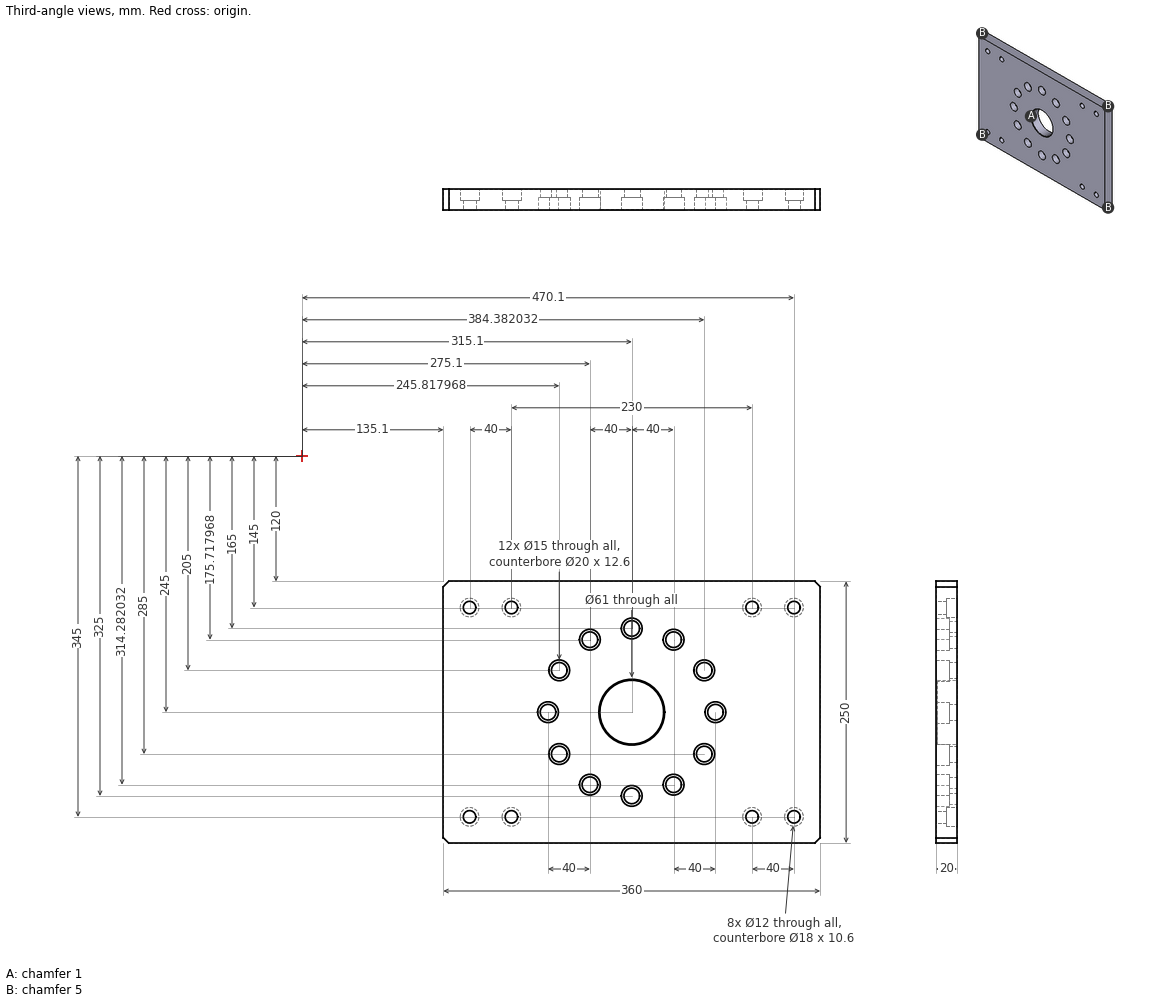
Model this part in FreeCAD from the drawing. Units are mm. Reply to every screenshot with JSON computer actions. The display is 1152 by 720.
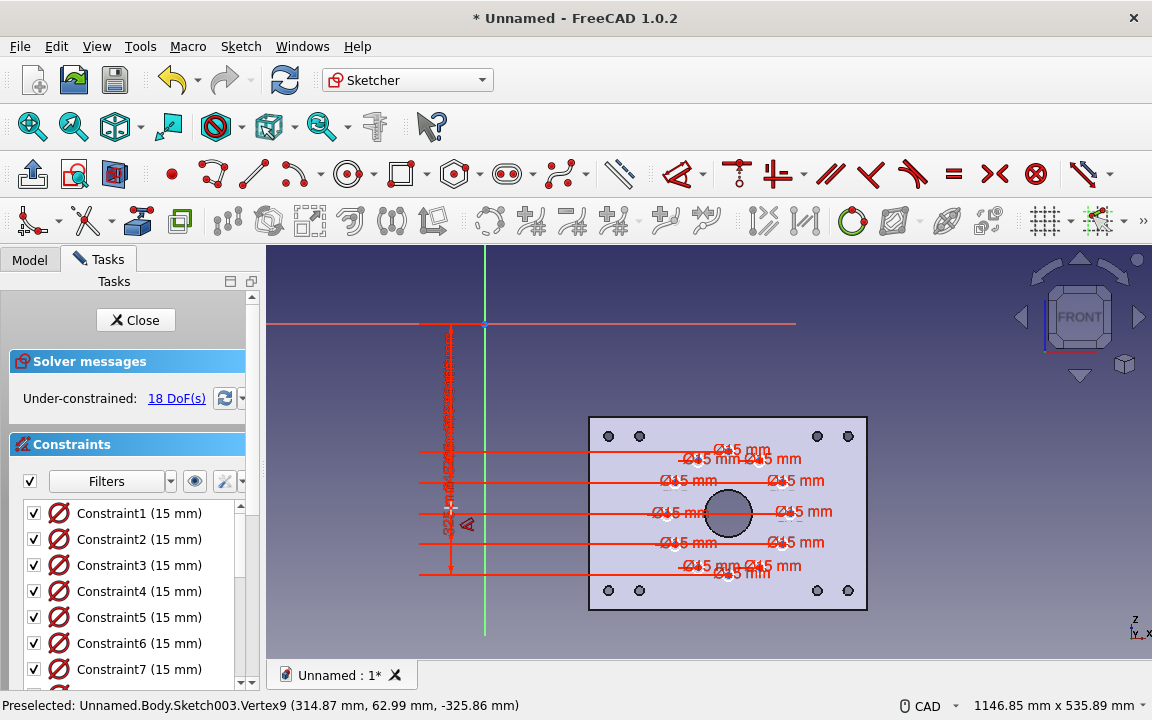
{"action": "left_click", "coordinate": [675, 545]}
{"action": "left_click", "coordinate": [451, 485]}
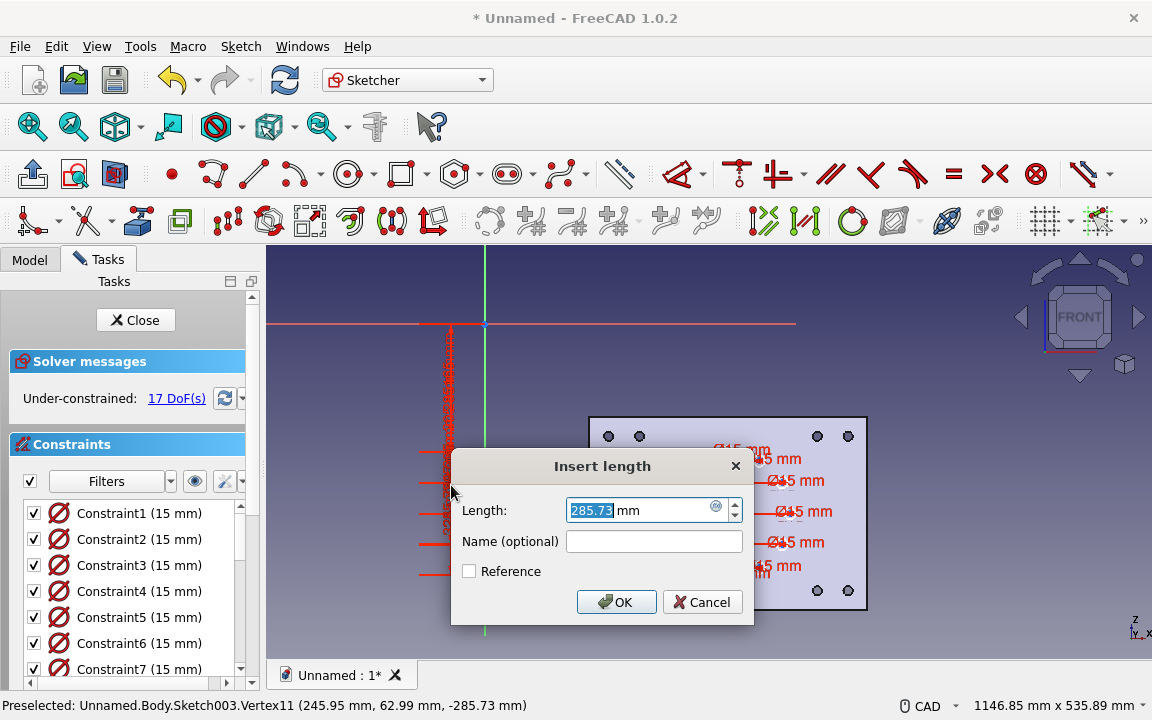
{"action": "type", "text": "285"}
{"action": "key", "text": "Return"}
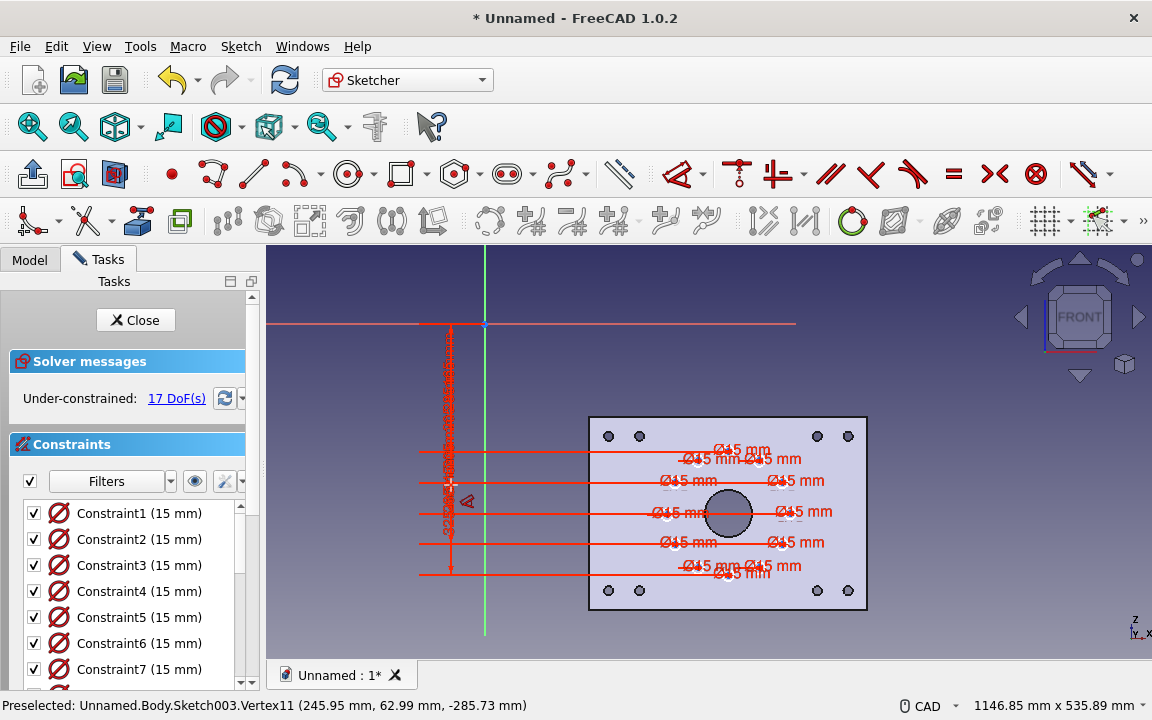
{"action": "left_click", "coordinate": [667, 515]}
{"action": "left_click", "coordinate": [701, 420]}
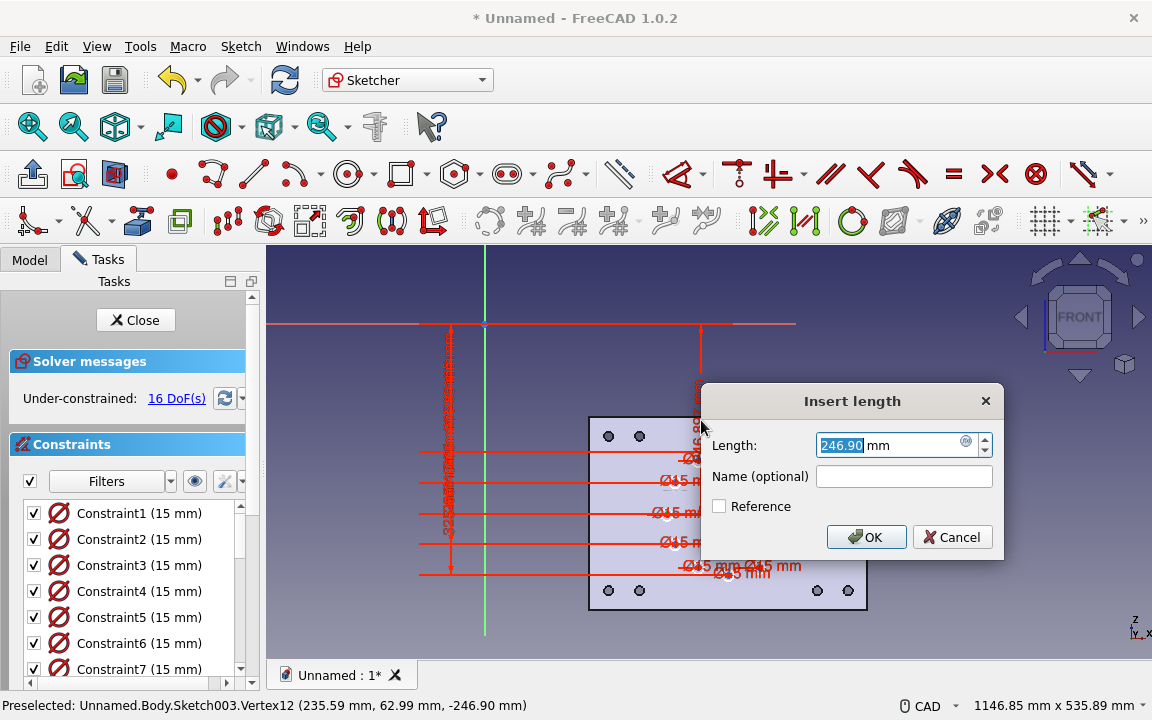
{"action": "type", "text": "245"}
{"action": "key", "text": "Return"}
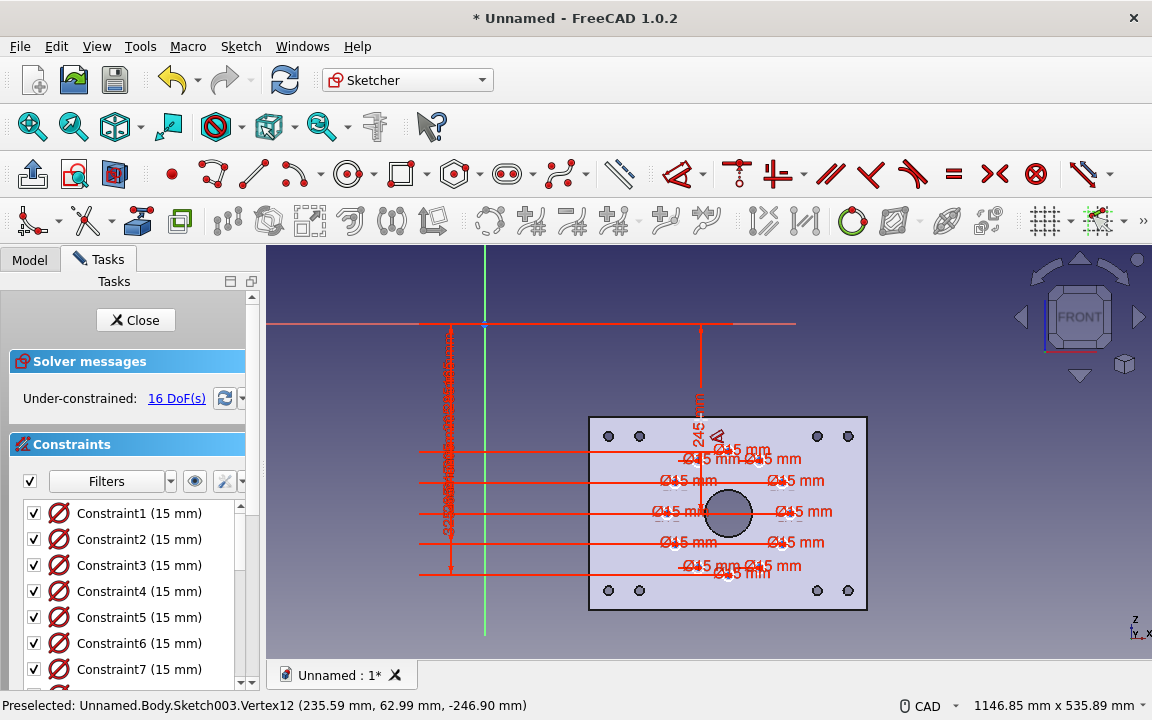
{"action": "scroll", "coordinate": [698, 461], "scroll_direction": "up", "scroll_amount": 2}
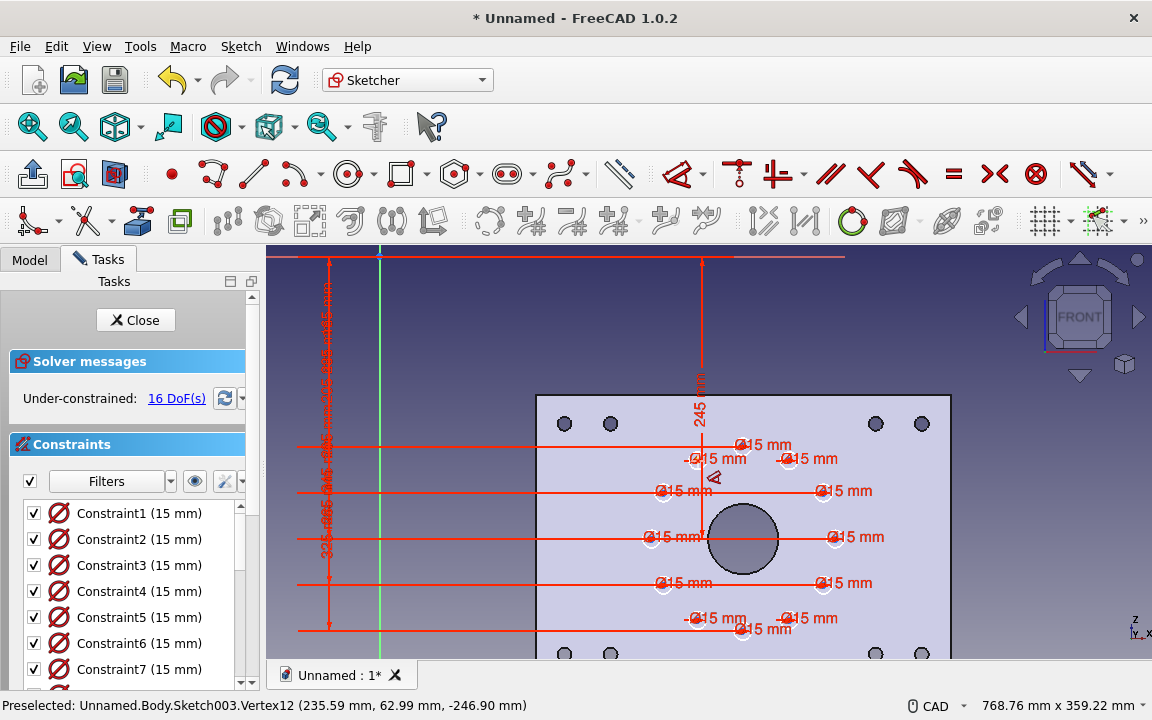
{"action": "left_click", "coordinate": [698, 461]}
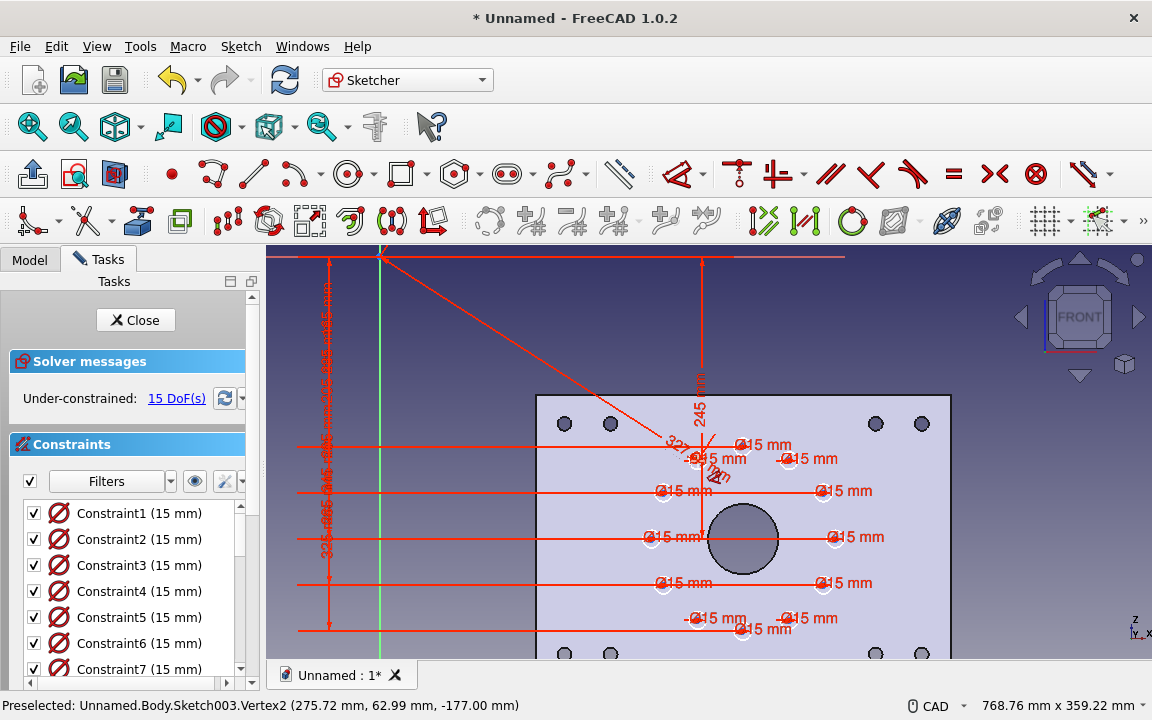
{"action": "left_click", "coordinate": [743, 447]}
{"action": "left_click", "coordinate": [720, 495]}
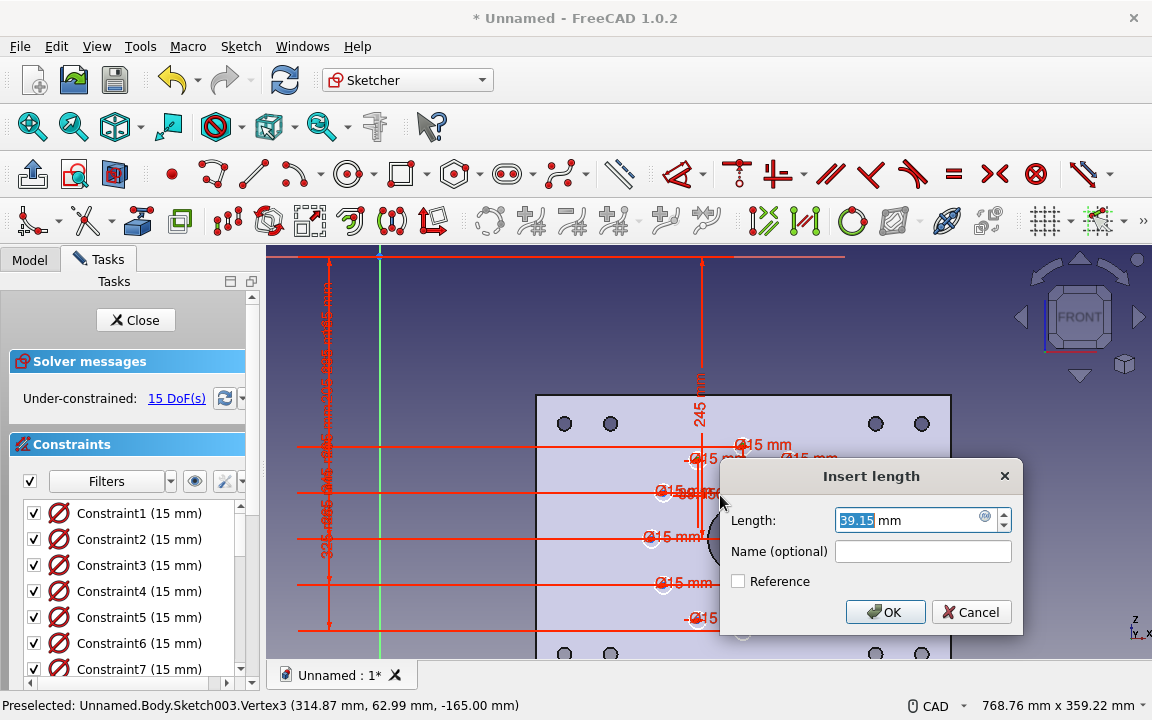
{"action": "type", "text": "40"}
{"action": "key", "text": "Return"}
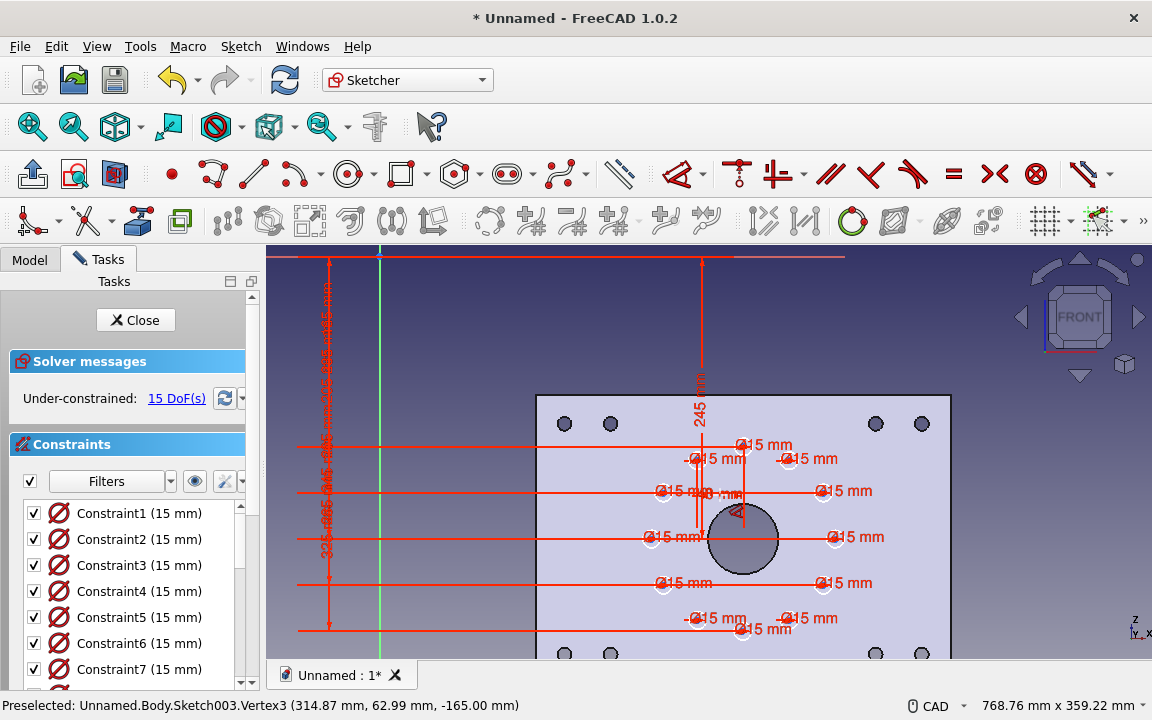
{"action": "left_click", "coordinate": [744, 447]}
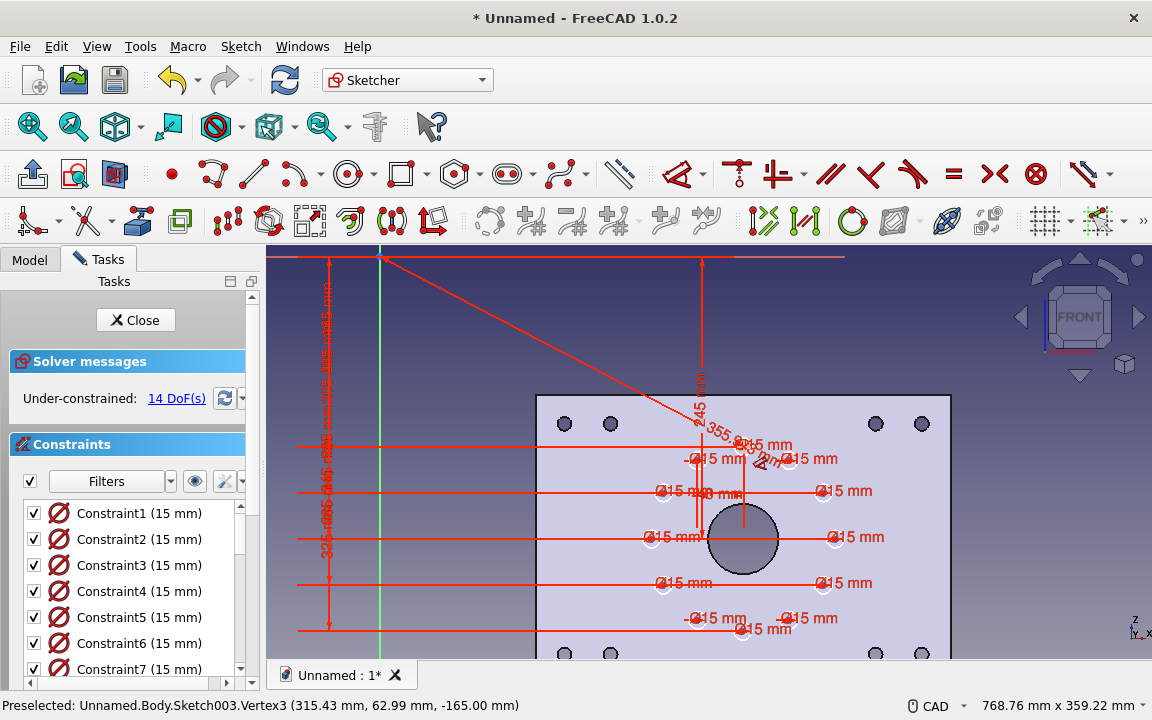
{"action": "left_click", "coordinate": [789, 461]}
{"action": "left_click", "coordinate": [777, 413]}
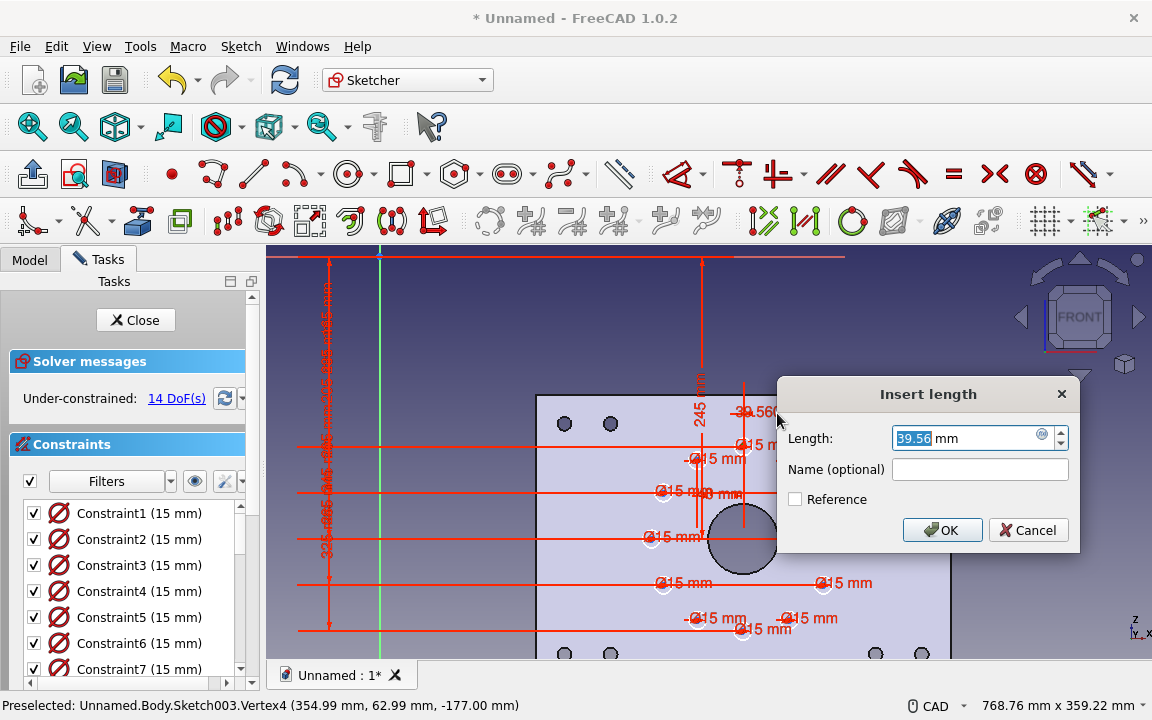
{"action": "type", "text": "40"}
{"action": "key", "text": "Return"}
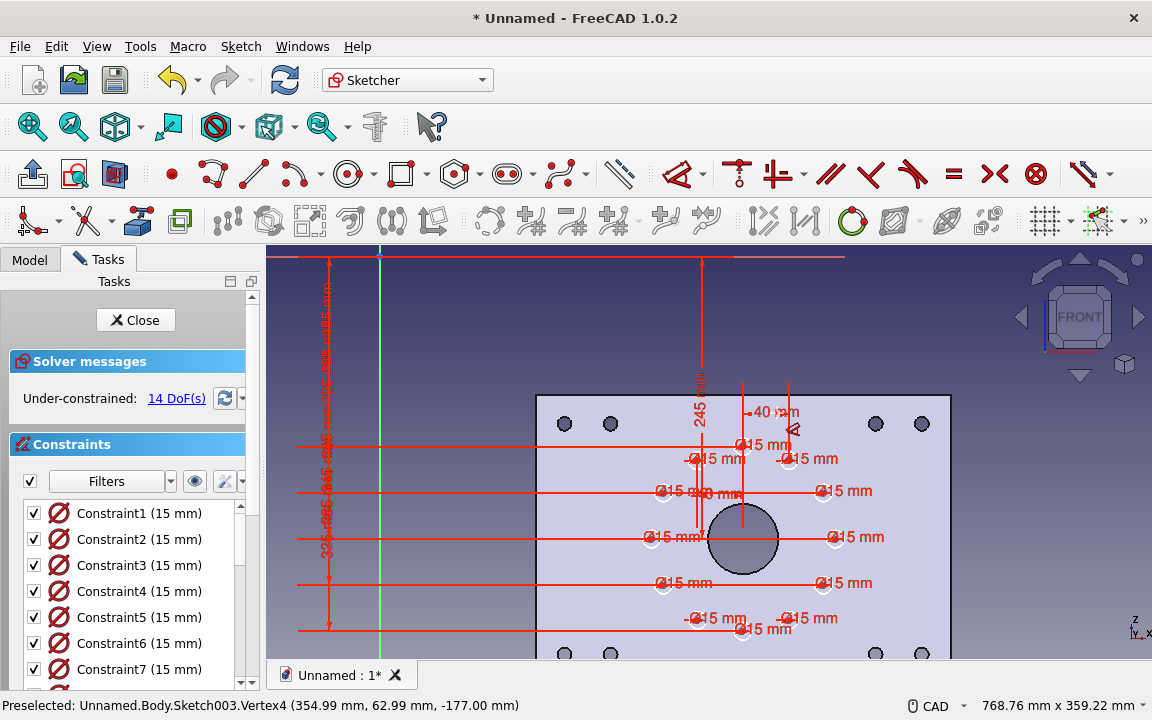
{"action": "left_click", "coordinate": [789, 461]}